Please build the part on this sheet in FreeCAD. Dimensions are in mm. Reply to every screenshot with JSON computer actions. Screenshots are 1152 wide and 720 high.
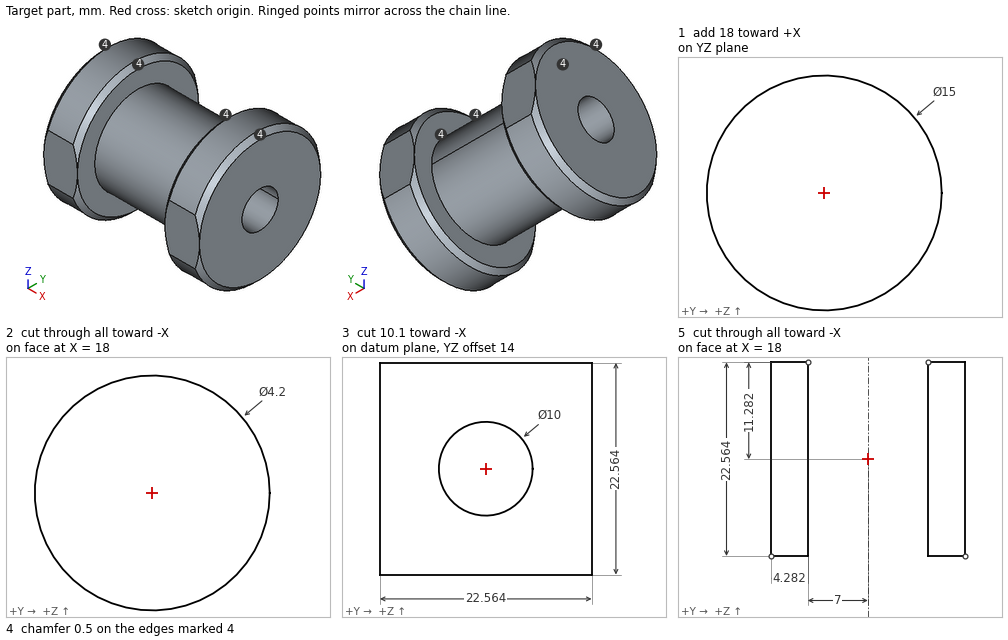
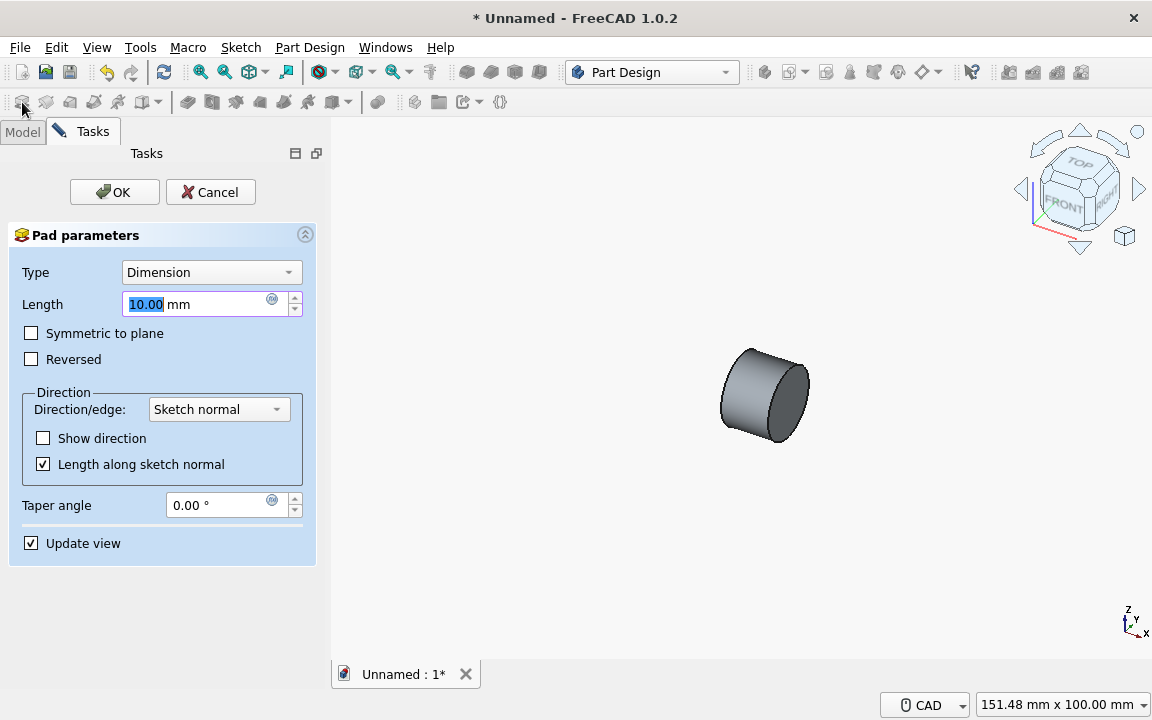
{"action": "type", "text": "18"}
{"action": "key", "text": "Tab"}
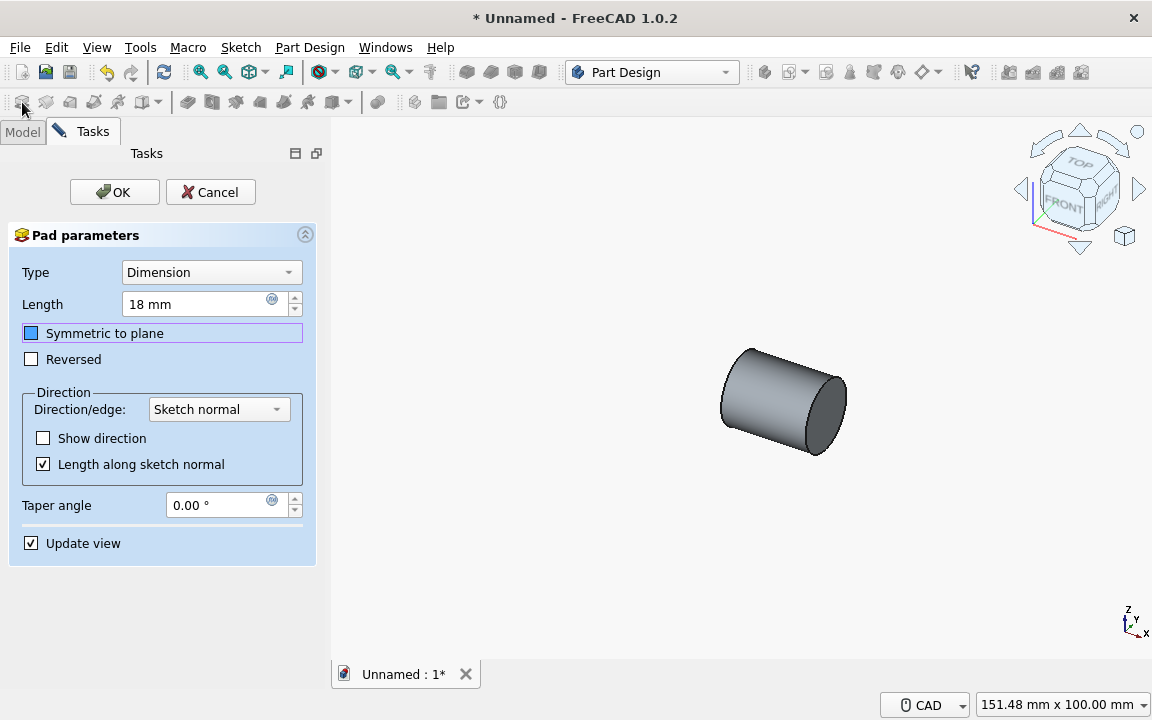
{"action": "left_click", "coordinate": [115, 192]}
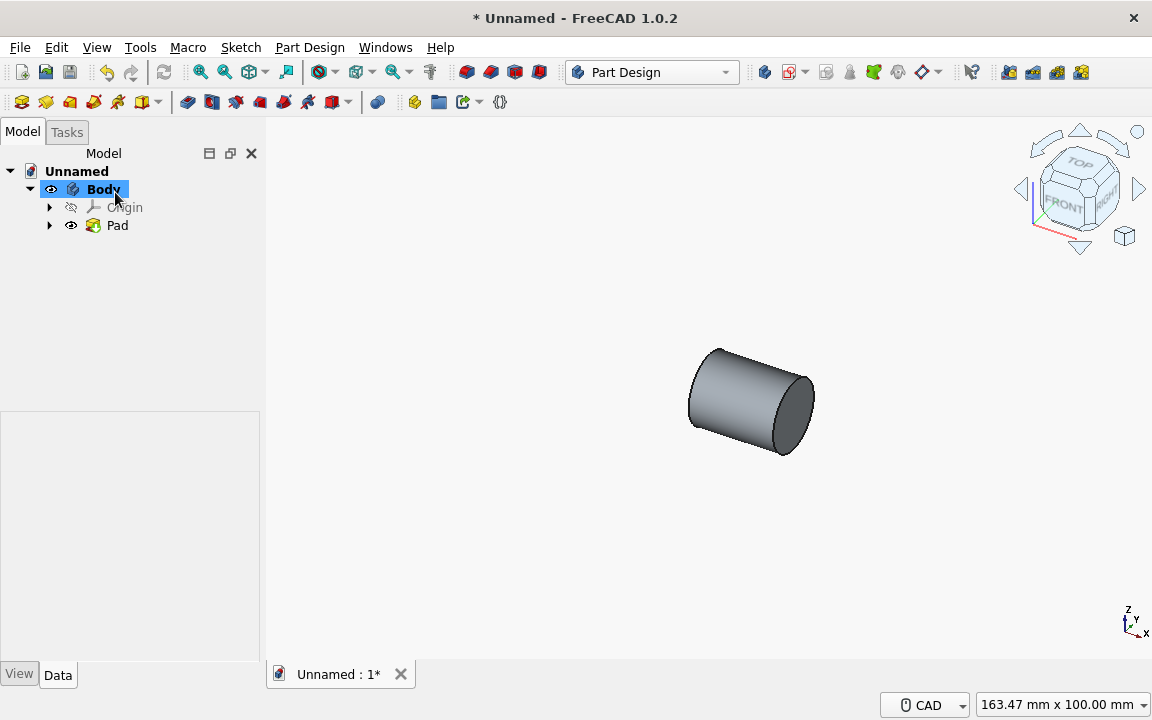
{"action": "left_click", "coordinate": [202, 72]}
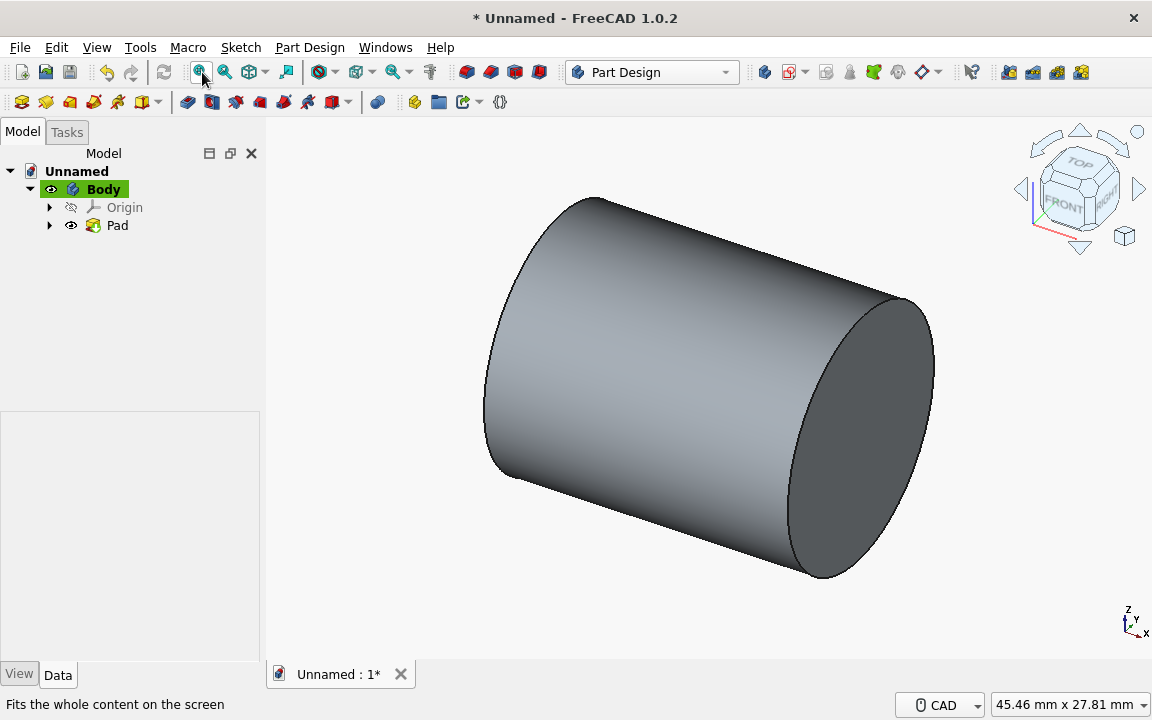
{"action": "left_click", "coordinate": [861, 437]}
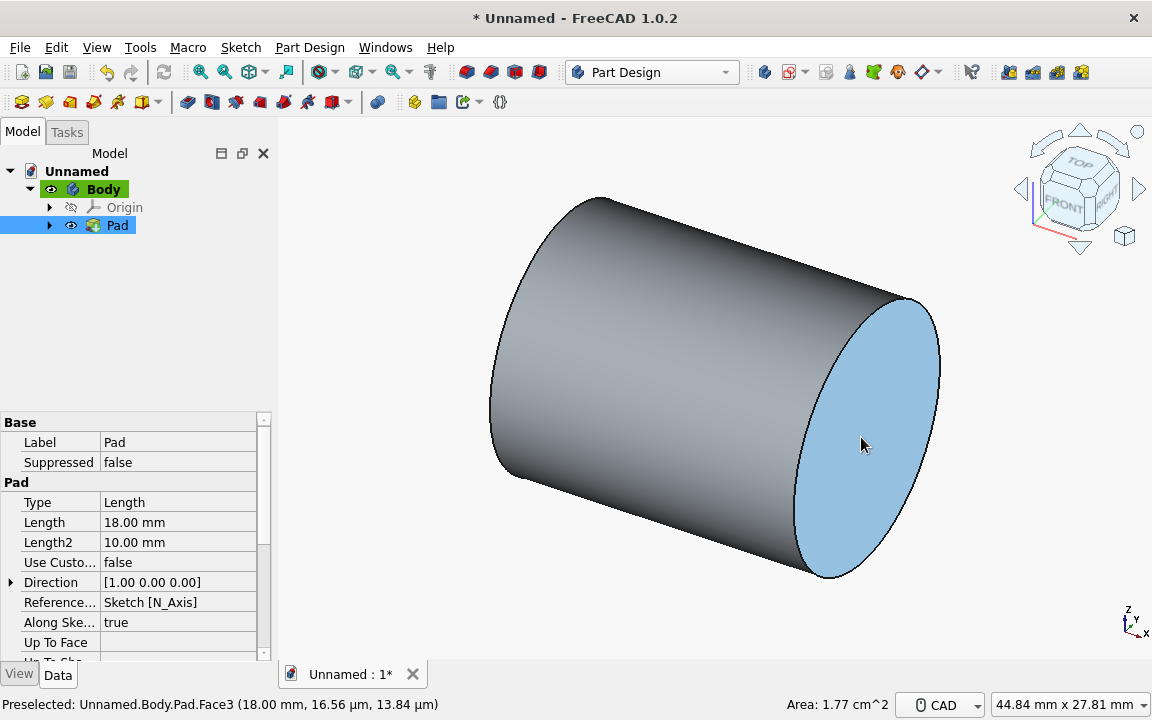
{"action": "left_click", "coordinate": [790, 72]}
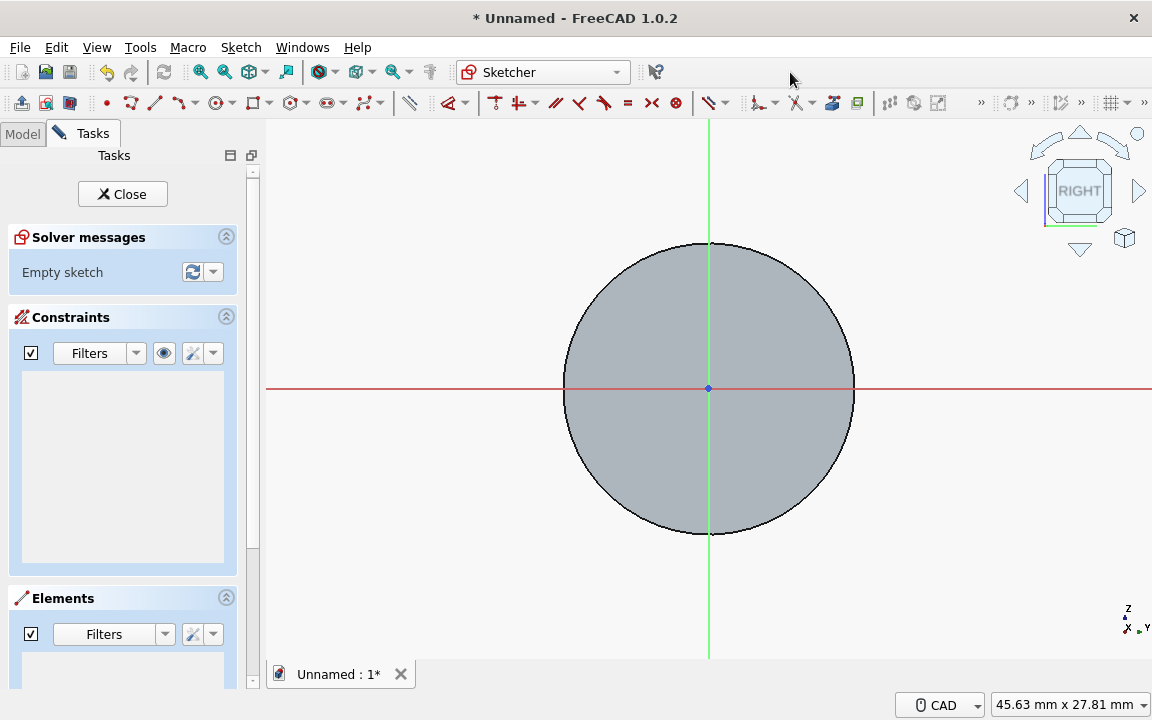
{"action": "scroll", "coordinate": [731, 389], "scroll_direction": "up", "scroll_amount": 7}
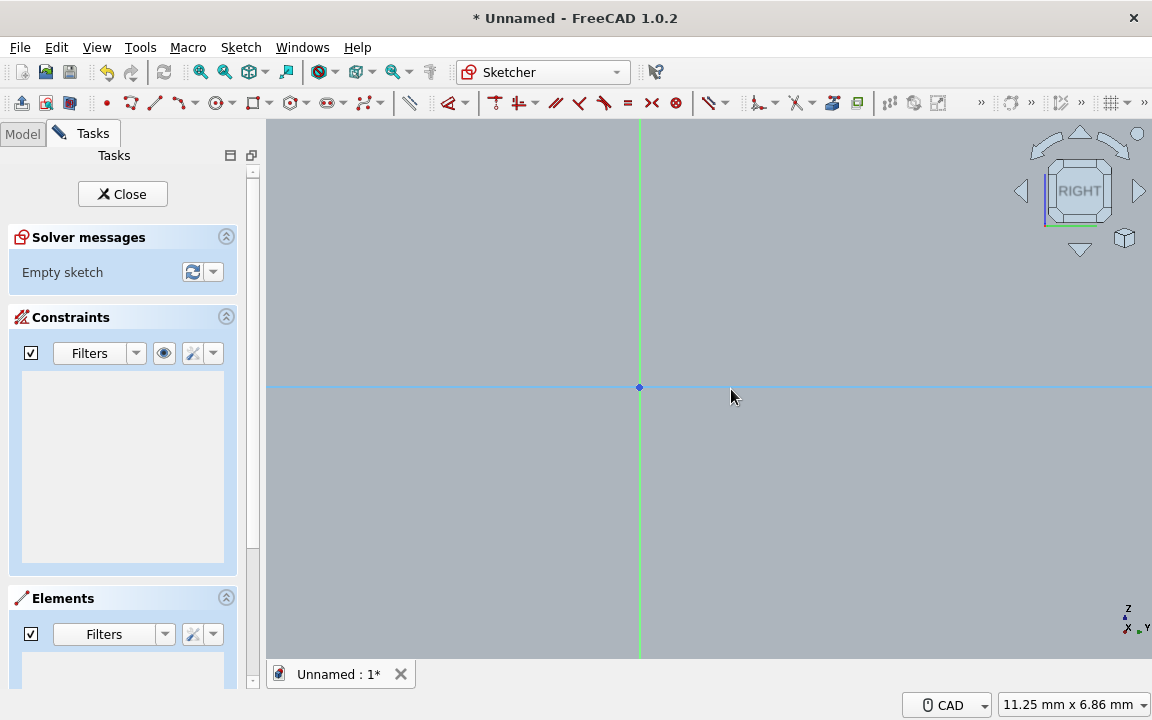
{"action": "left_click", "coordinate": [216, 104]}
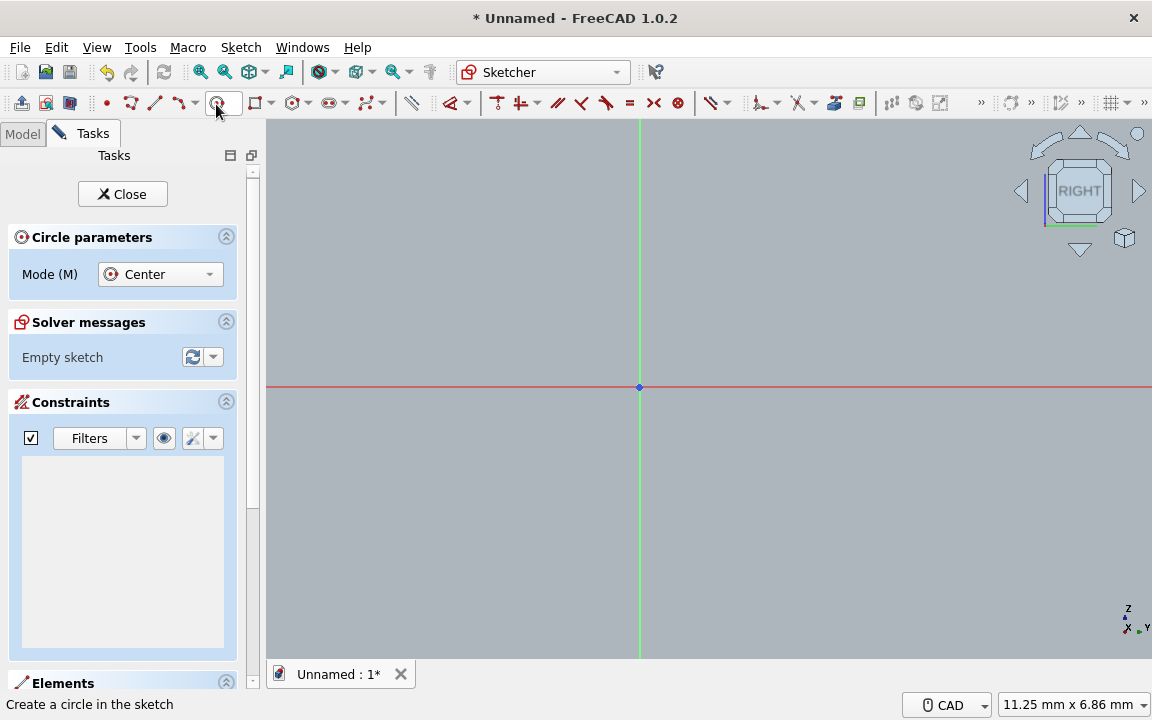
{"action": "left_click", "coordinate": [640, 387]}
{"action": "left_click", "coordinate": [757, 271]}
{"action": "key", "text": "Escape"}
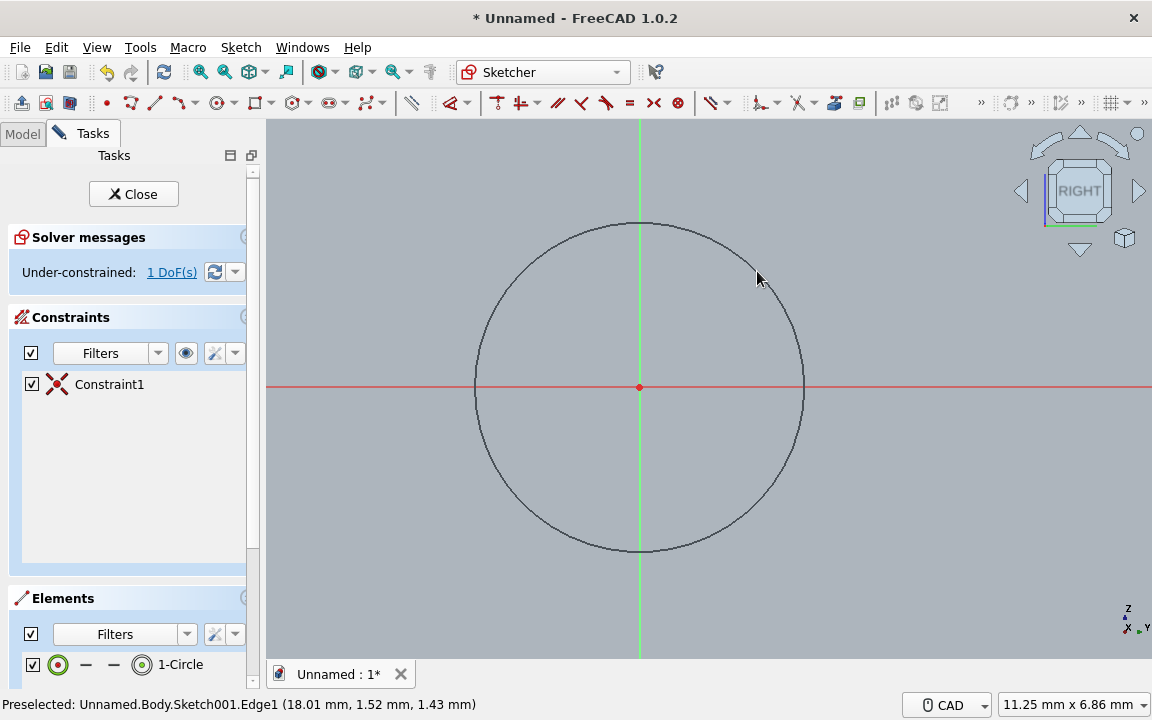
{"action": "left_click", "coordinate": [450, 104]}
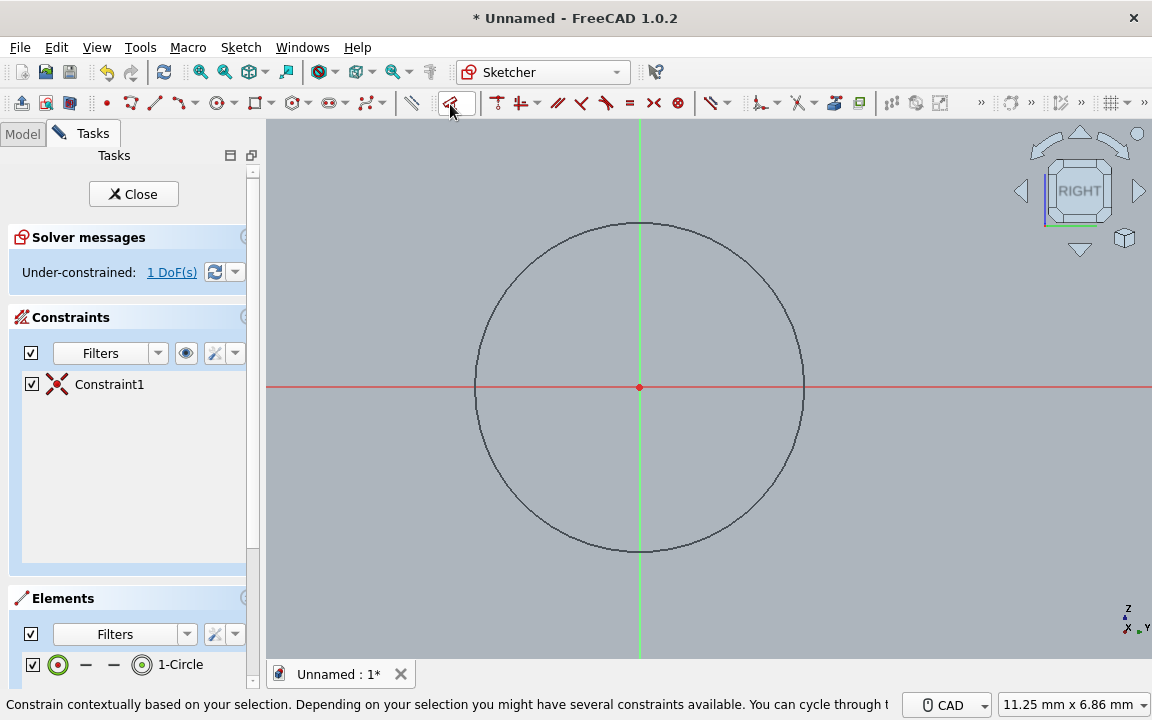
{"action": "left_click", "coordinate": [756, 271]}
{"action": "left_click", "coordinate": [779, 248]}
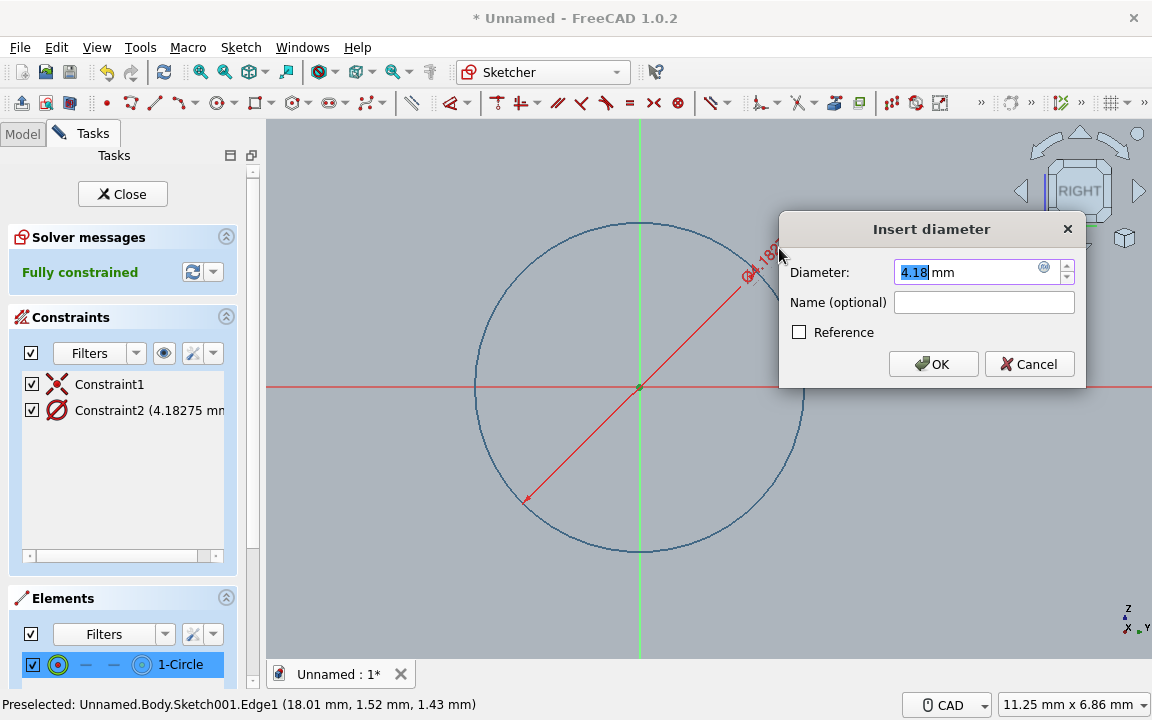
{"action": "type", "text": "4.2"}
{"action": "key", "text": "Return"}
{"action": "key", "text": "Escape"}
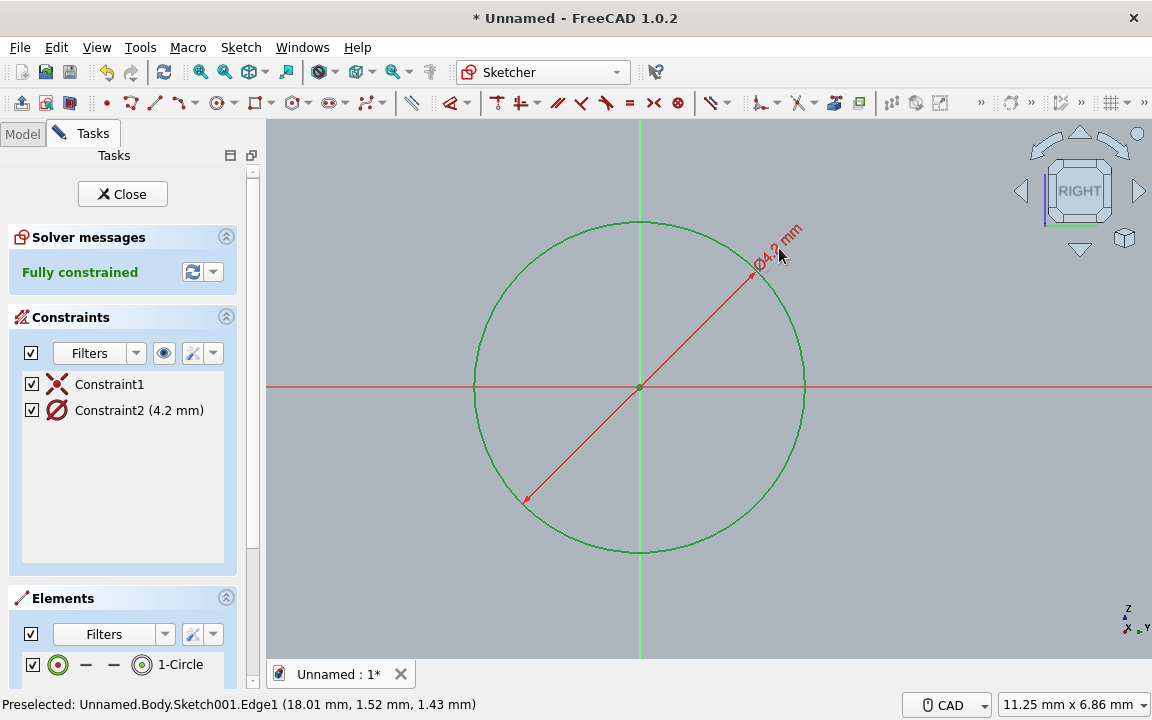
{"action": "left_click", "coordinate": [123, 194]}